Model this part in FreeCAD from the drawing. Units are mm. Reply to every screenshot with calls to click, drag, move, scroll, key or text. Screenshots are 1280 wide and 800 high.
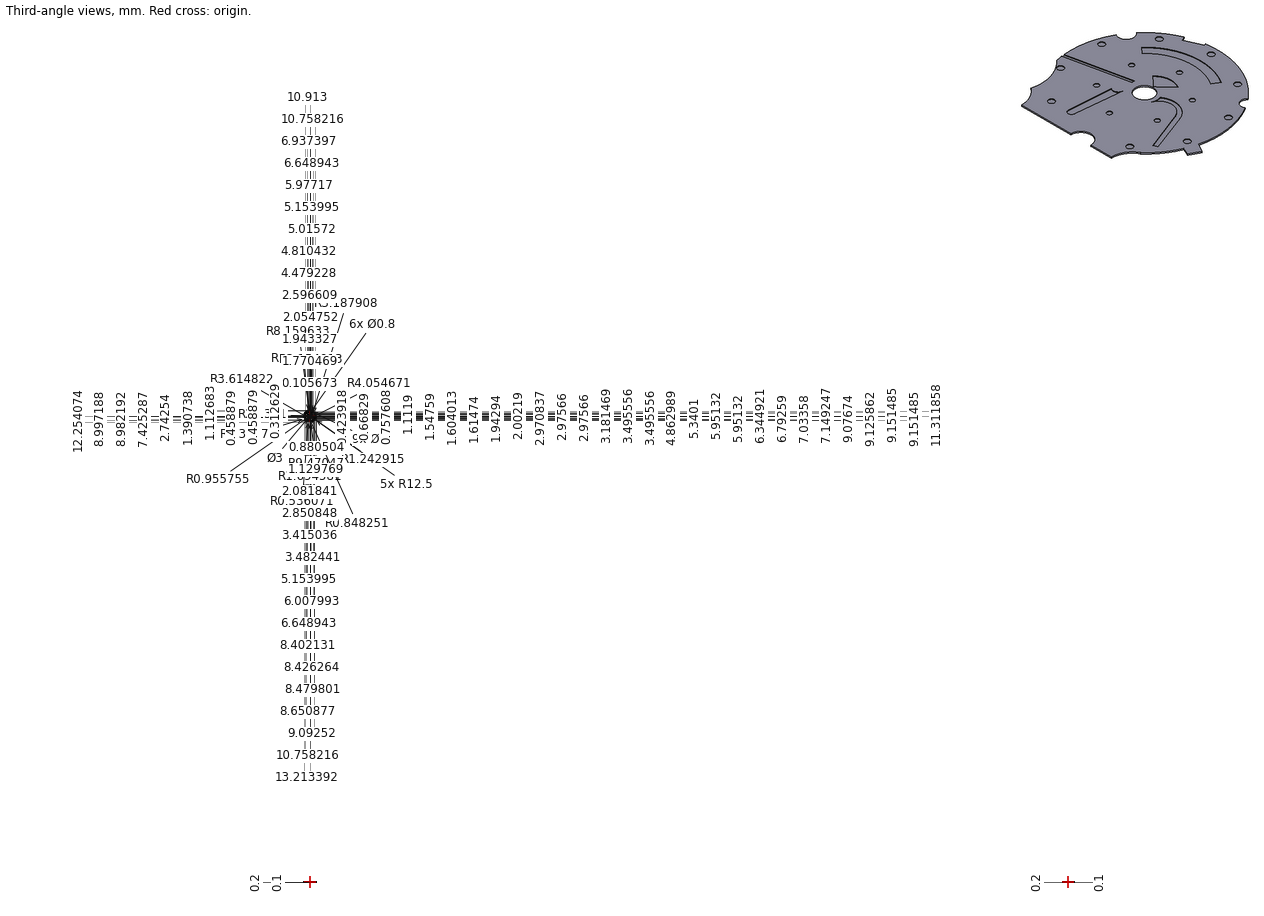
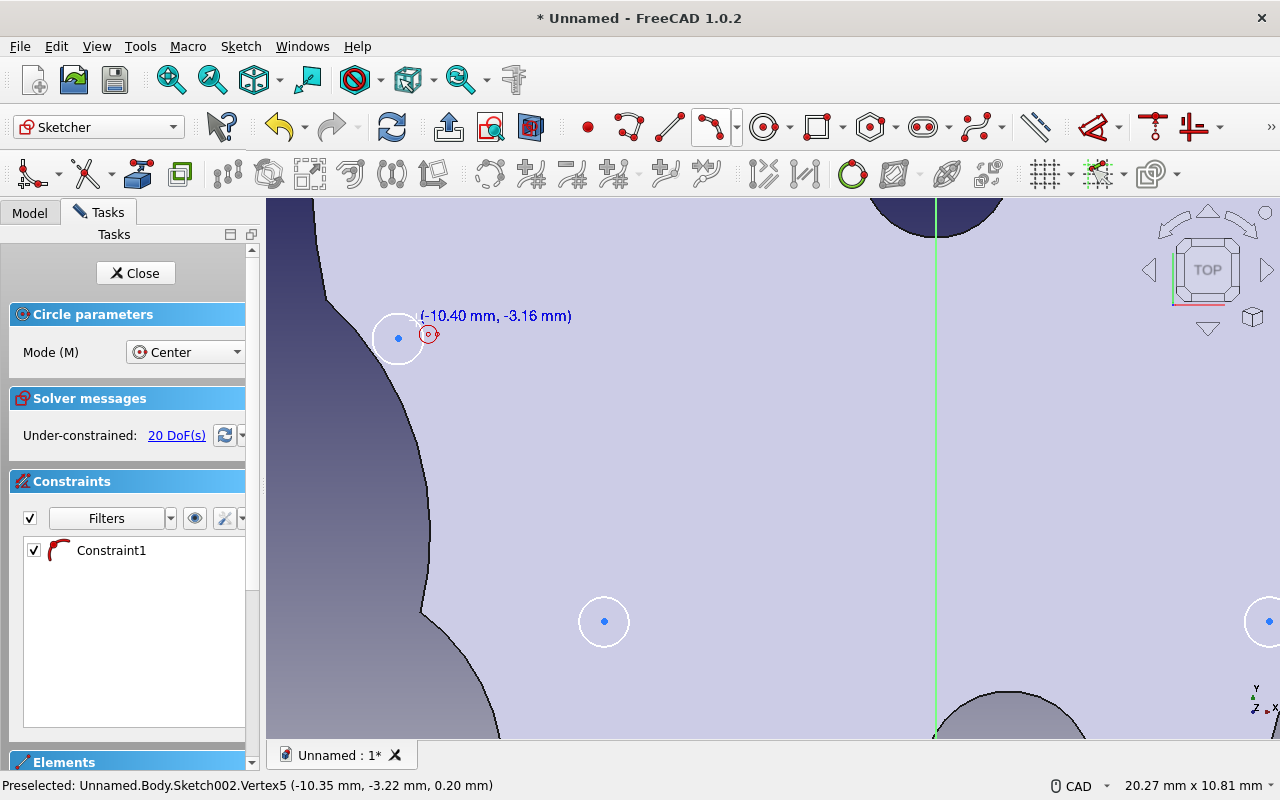
scroll(605, 624, down, 6)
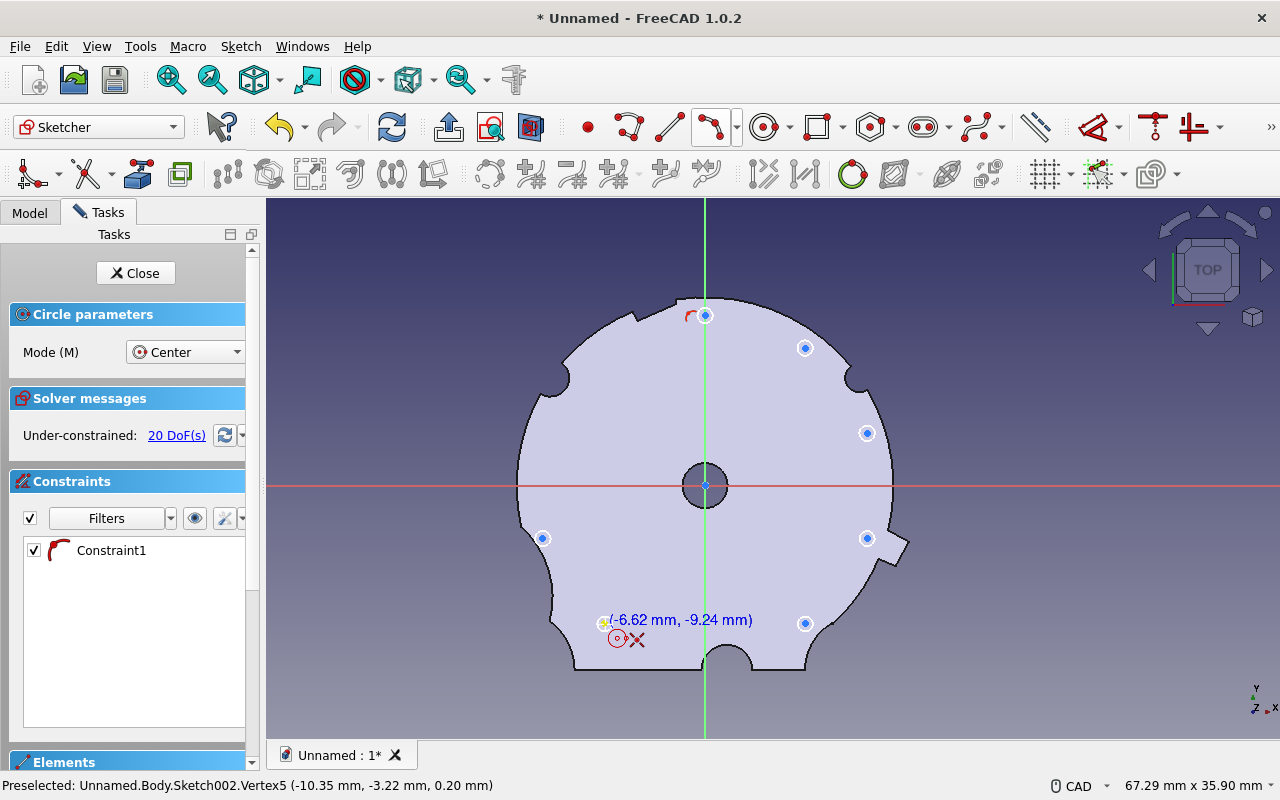
scroll(543, 433, up, 6)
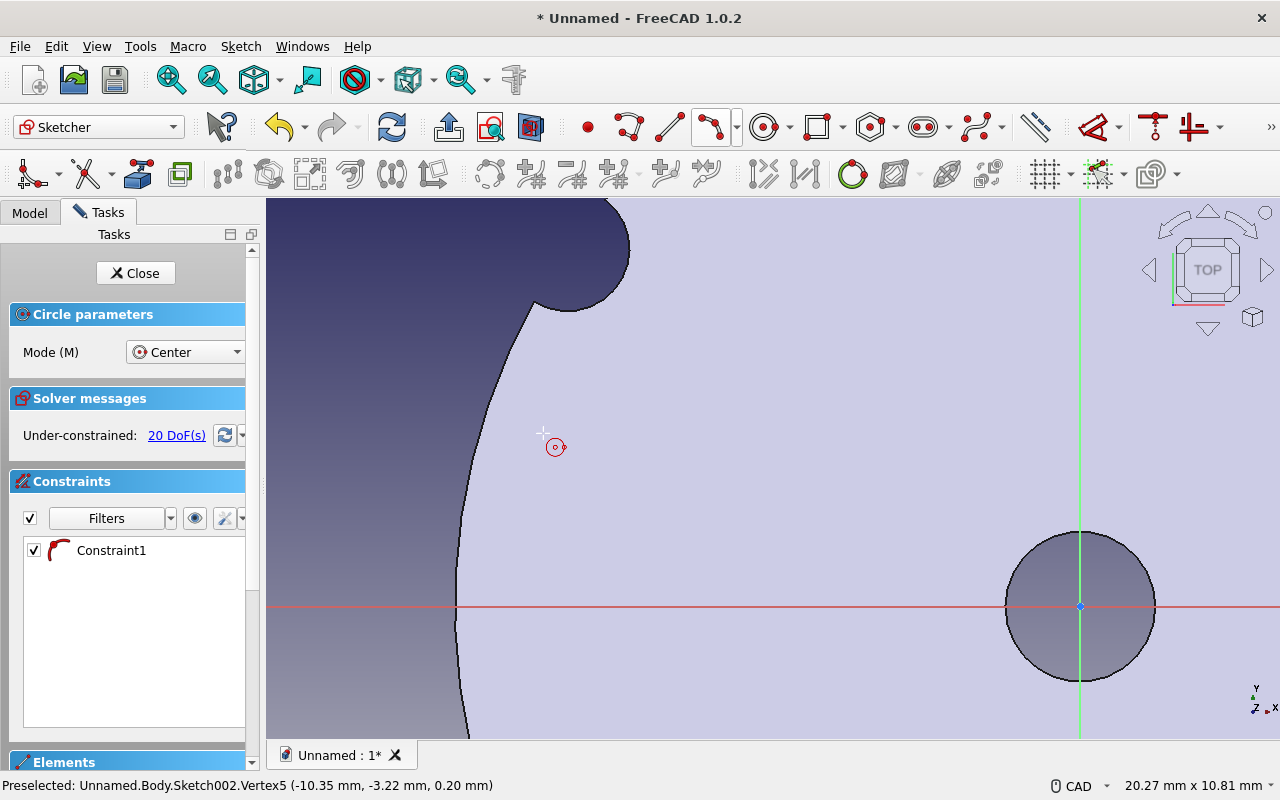
click(542, 432)
click(560, 414)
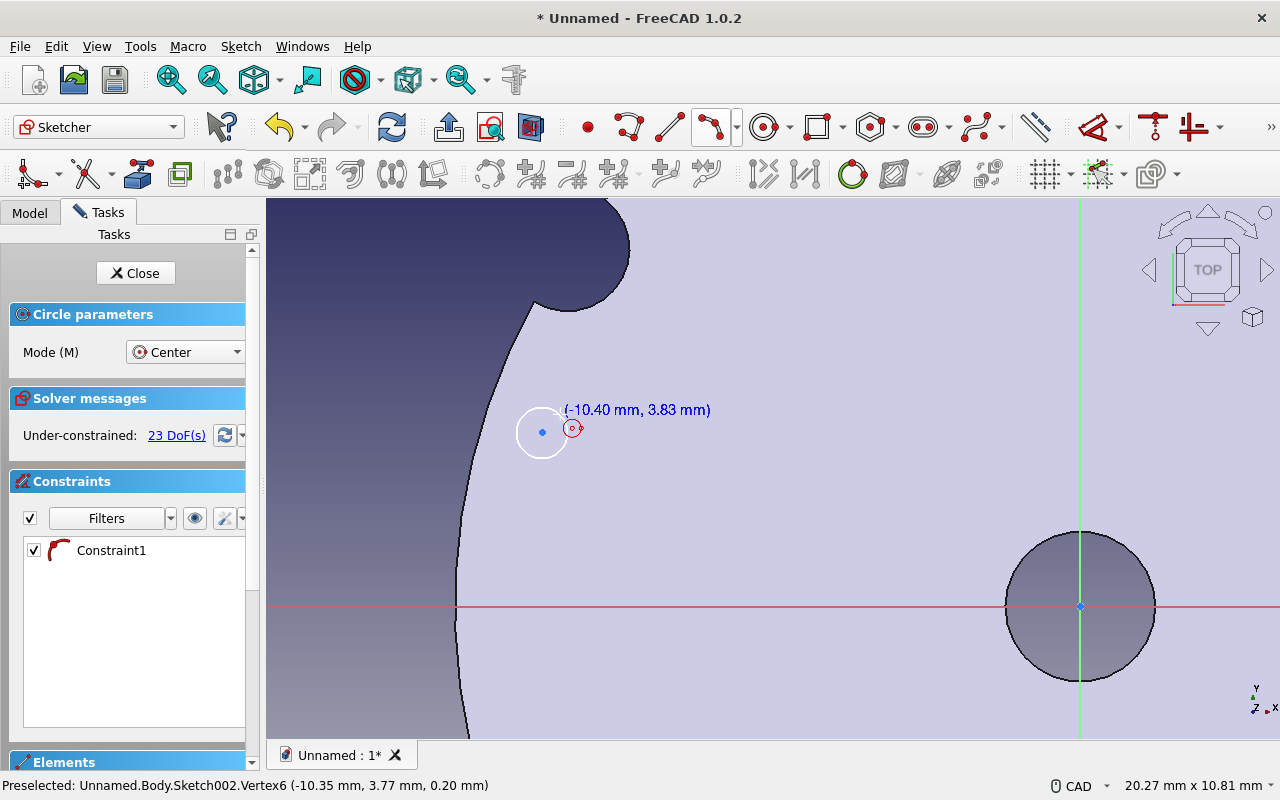
scroll(542, 432, down, 6)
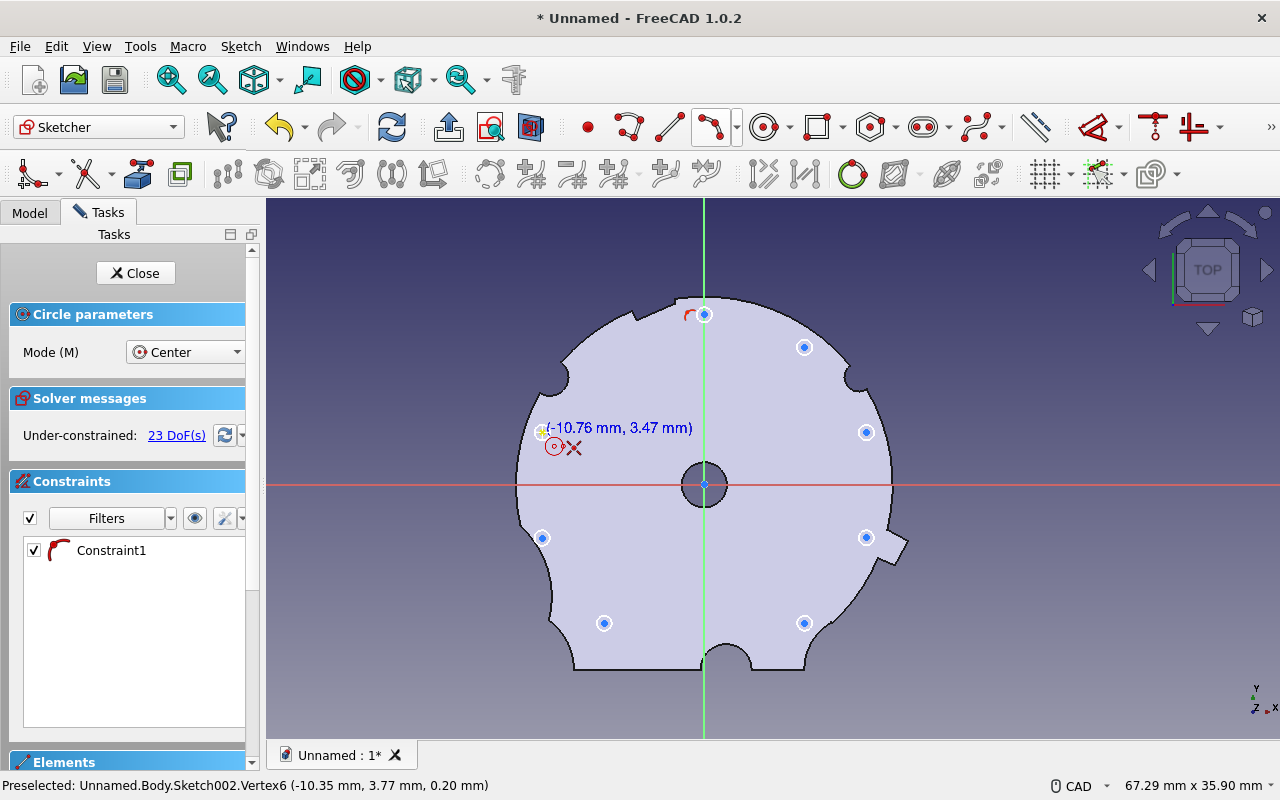
scroll(604, 347, up, 6)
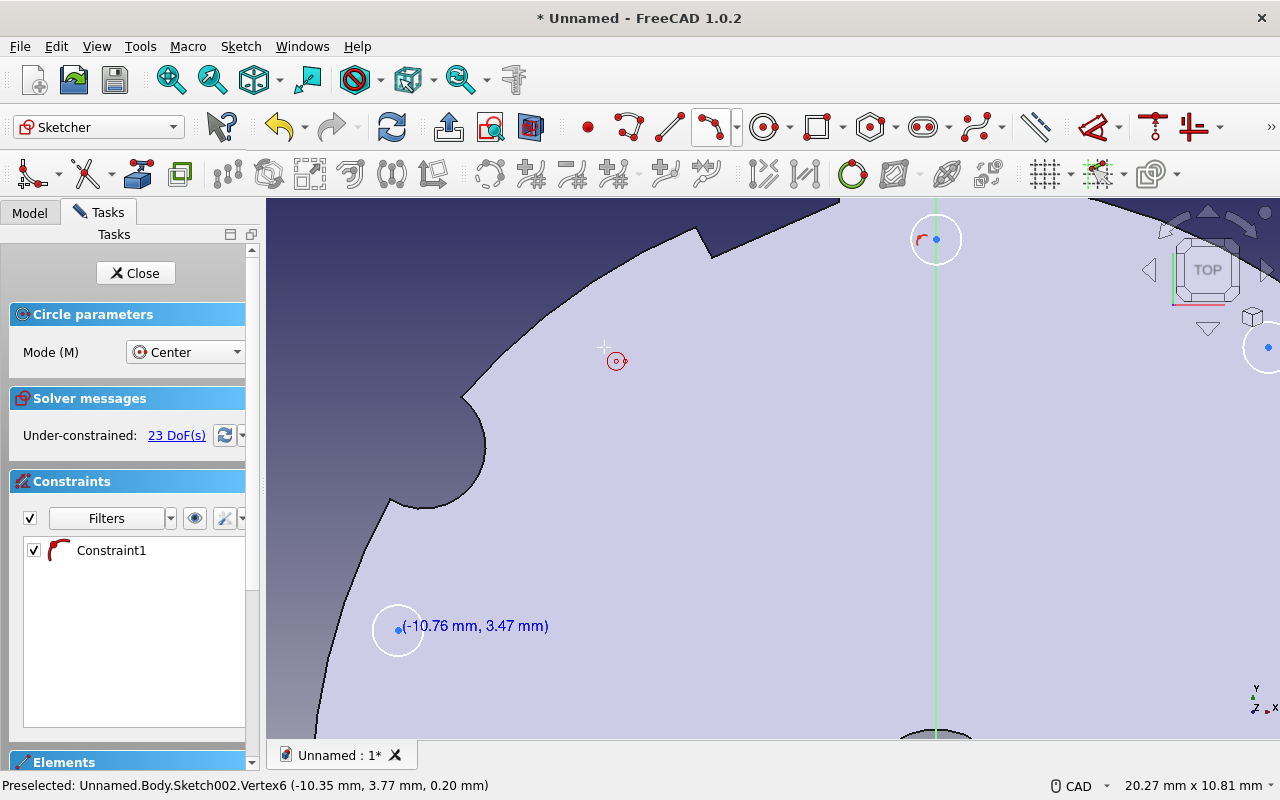
click(604, 346)
click(621, 329)
key(Escape)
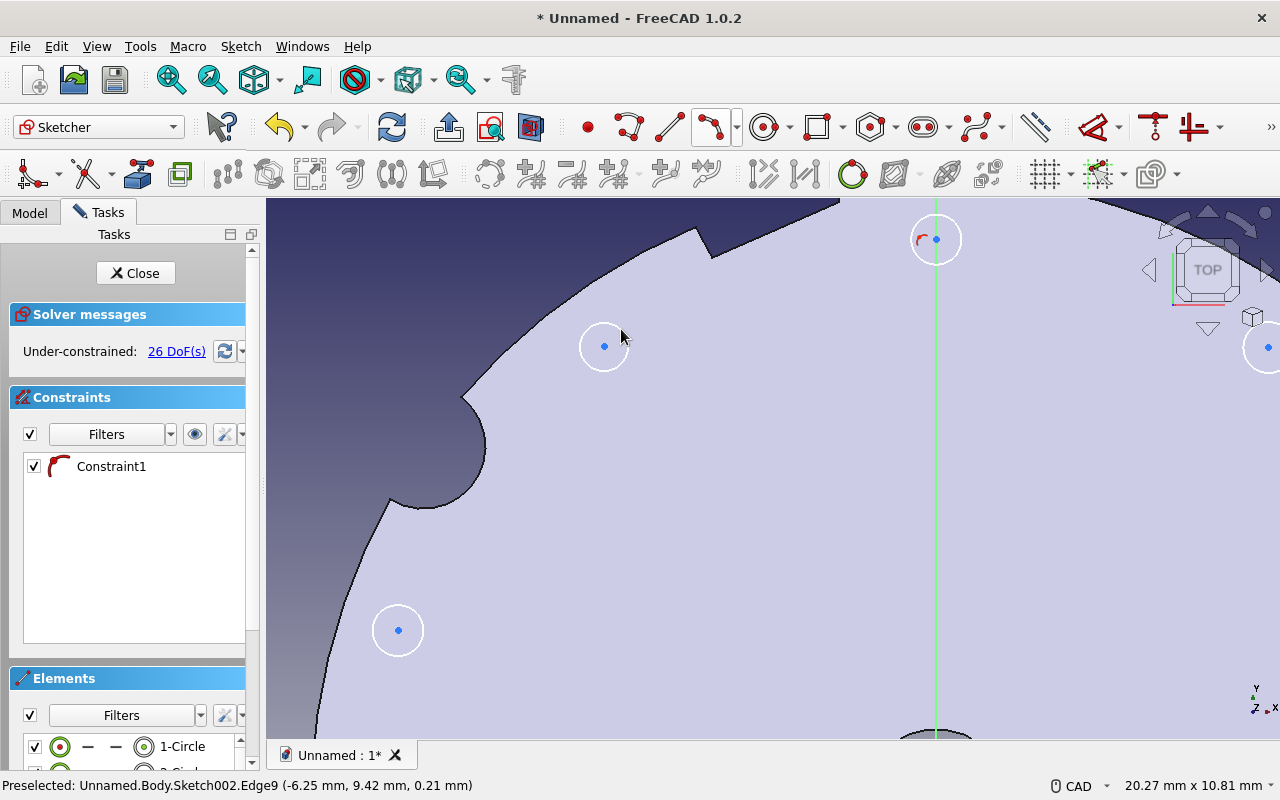
click(919, 257)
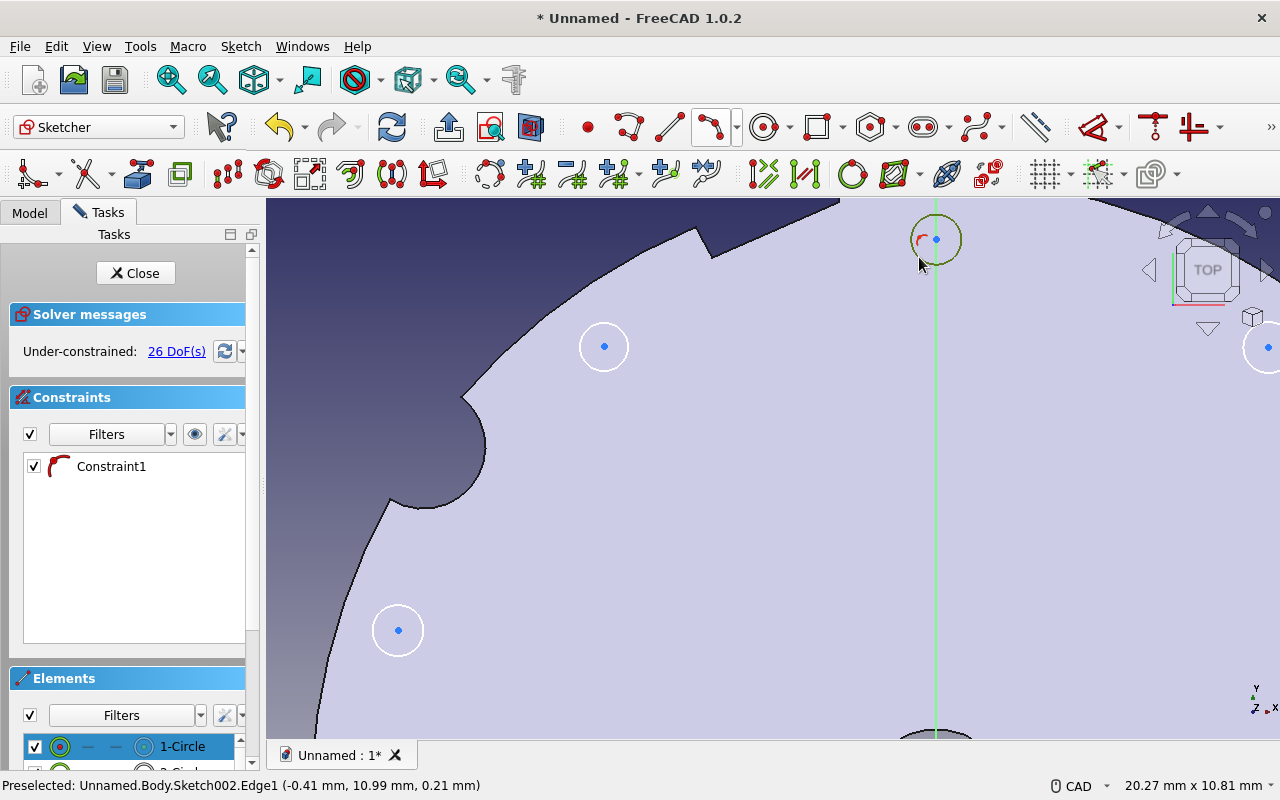
scroll(605, 347, down, 6)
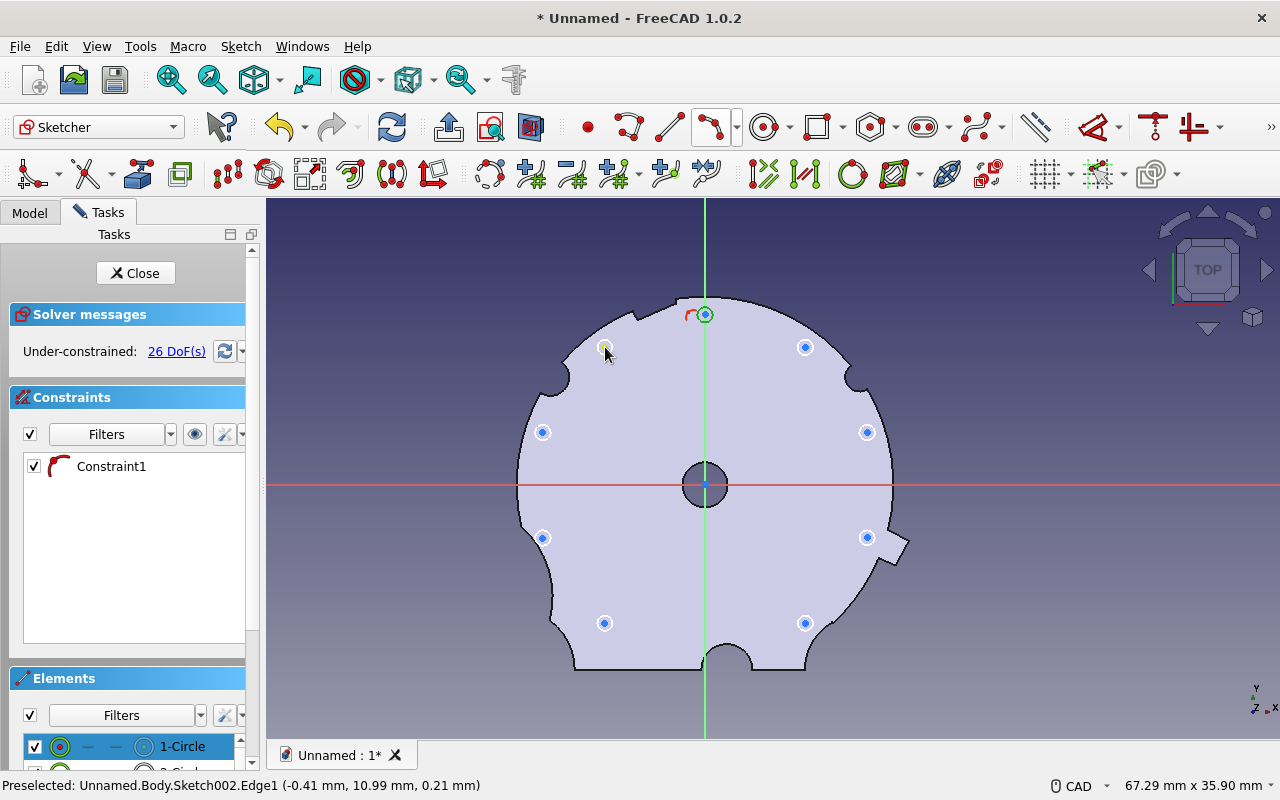
scroll(811, 342, up, 3)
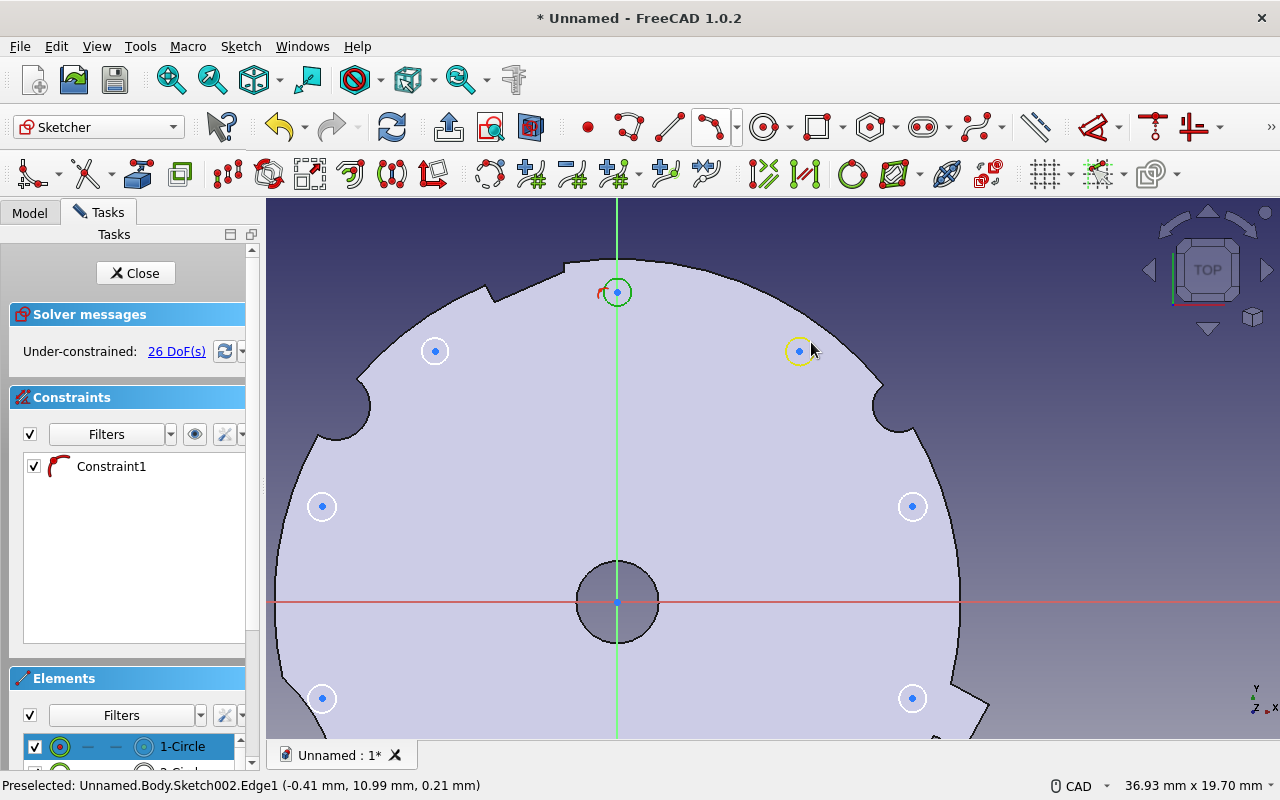
click(810, 342)